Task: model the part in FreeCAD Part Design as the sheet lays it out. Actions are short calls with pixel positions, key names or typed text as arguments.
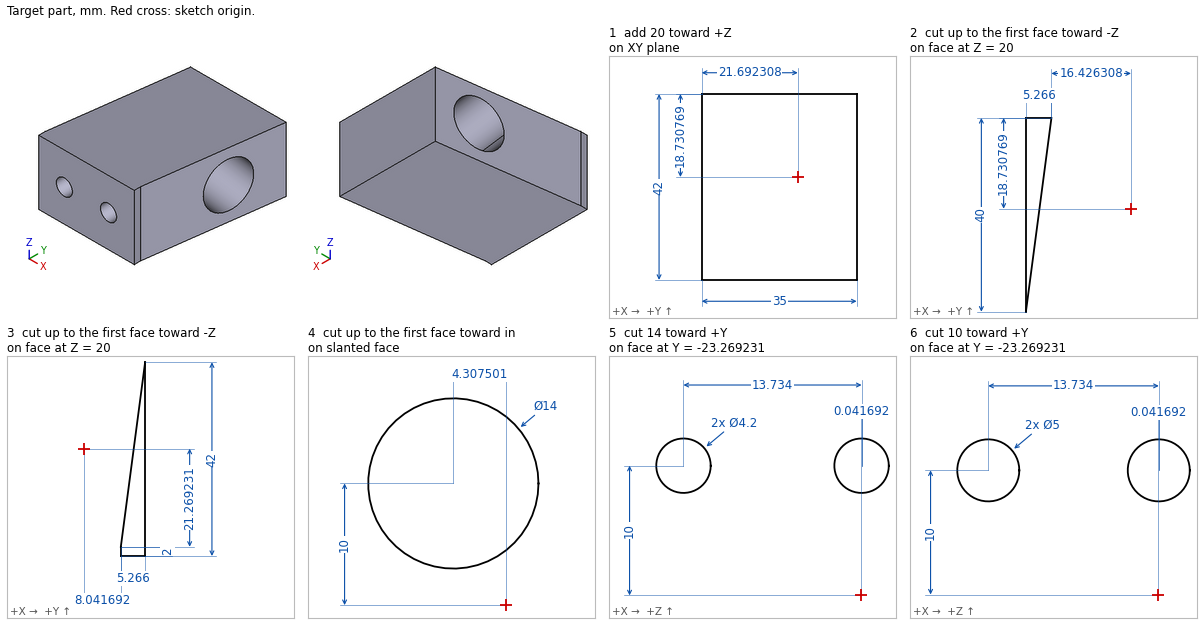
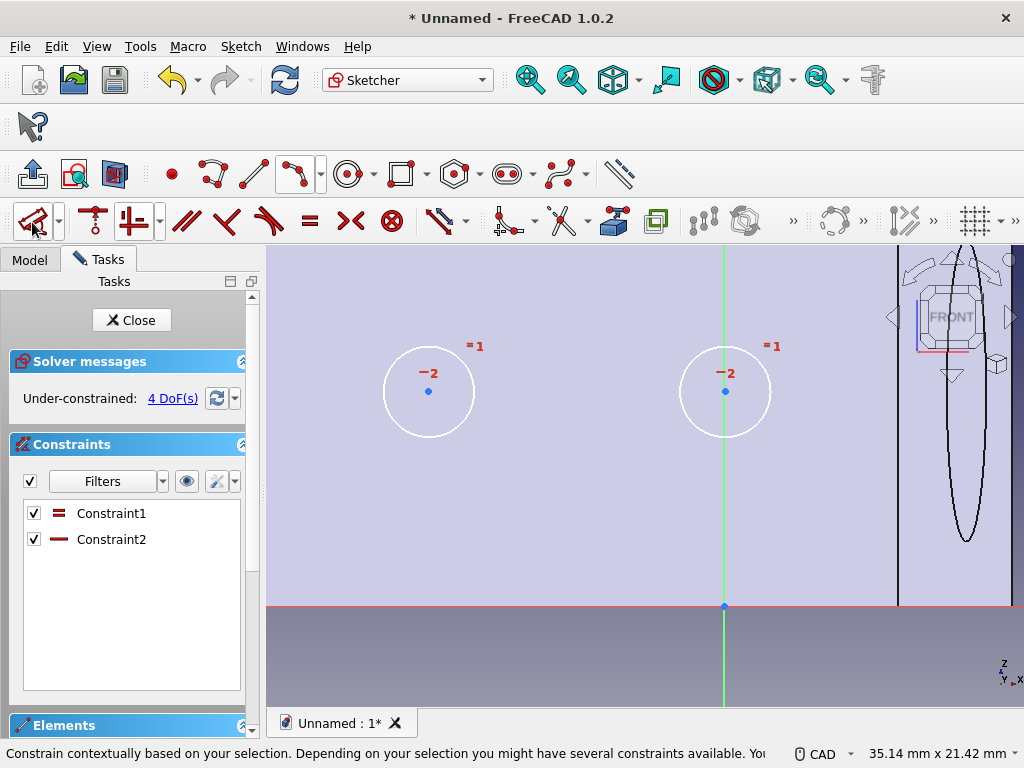
click(461, 360)
click(484, 337)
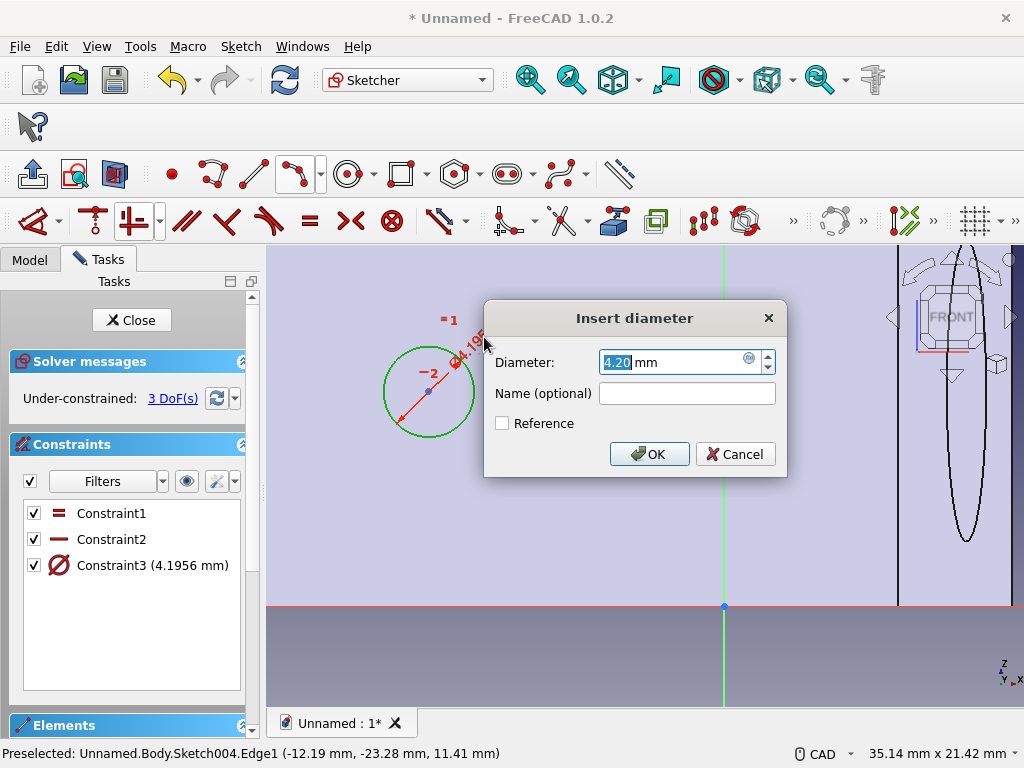
text(4.2)
key(Return)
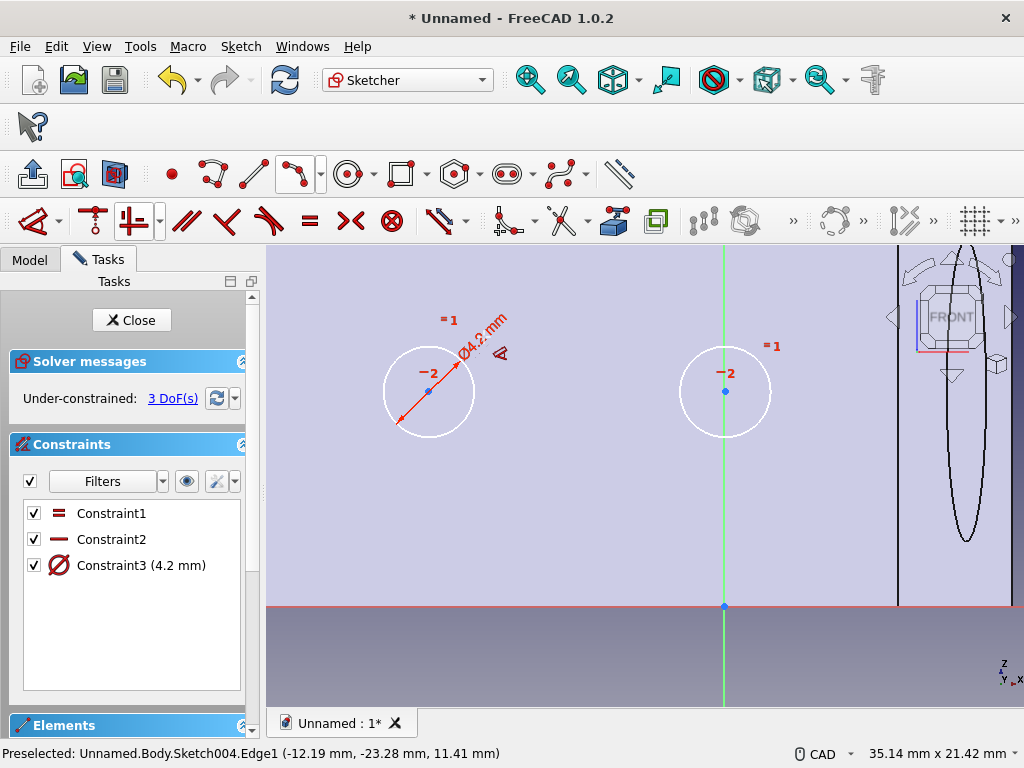
click(429, 392)
click(395, 499)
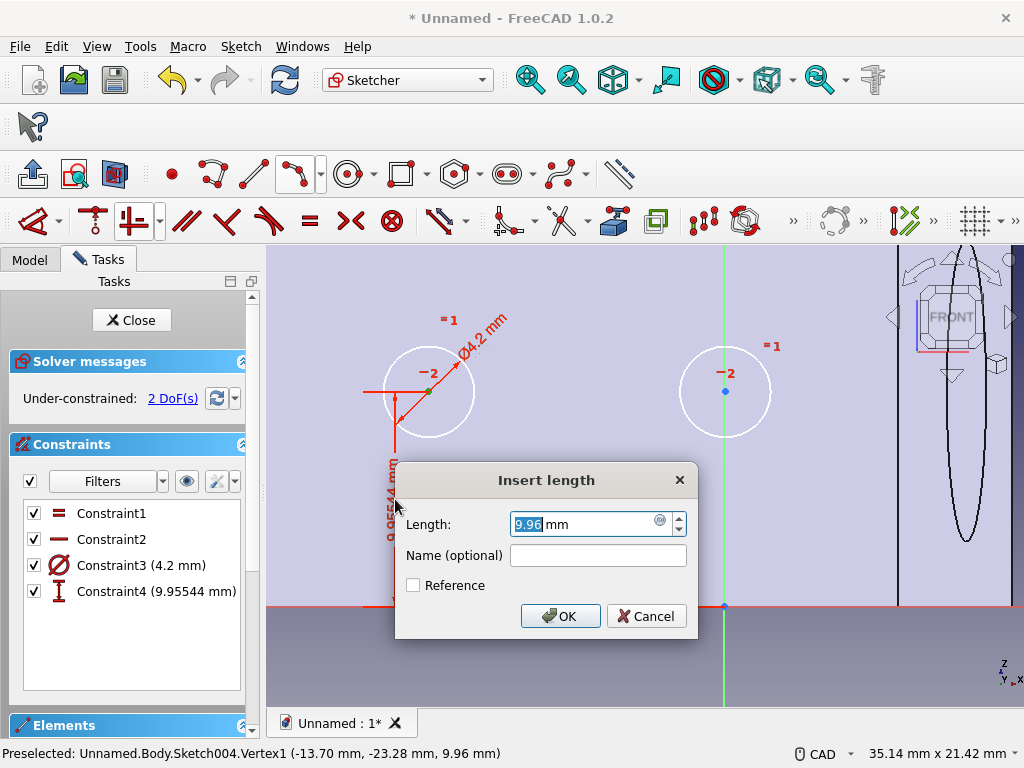
text(10)
key(Return)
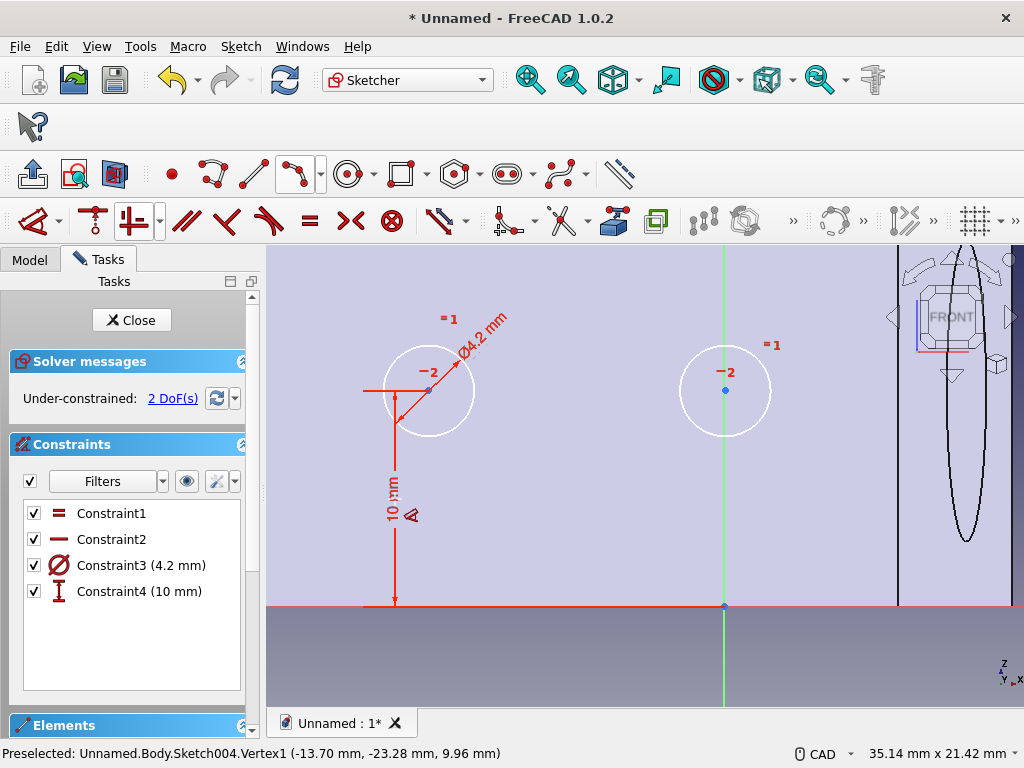
click(429, 391)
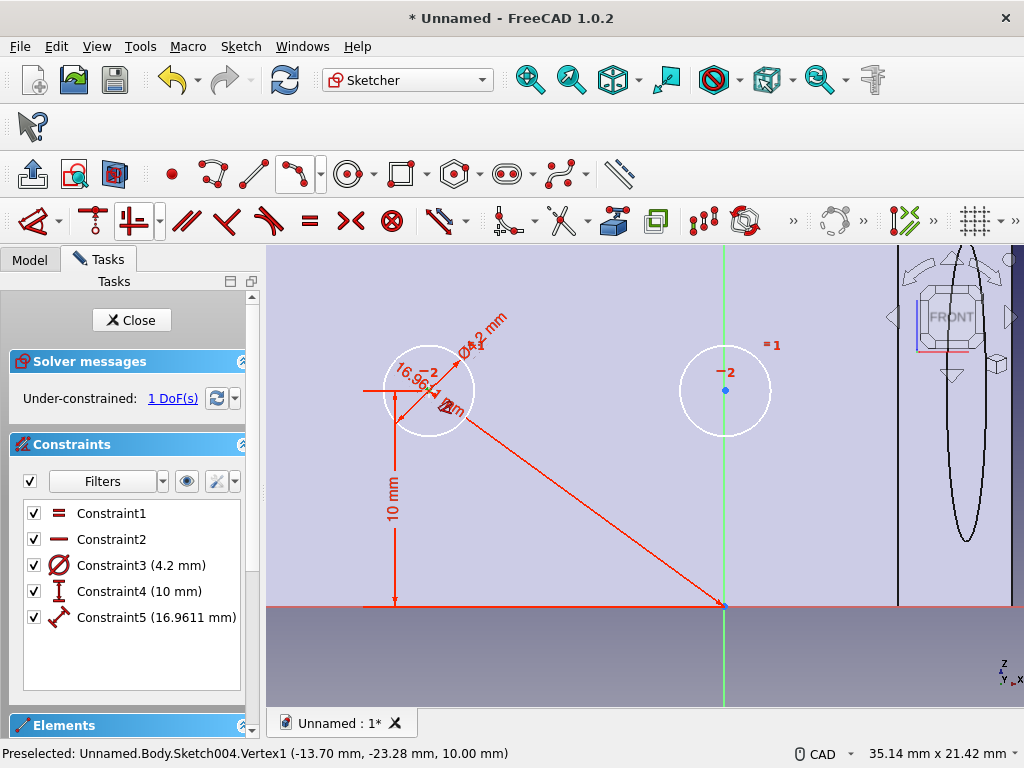
click(725, 391)
click(577, 357)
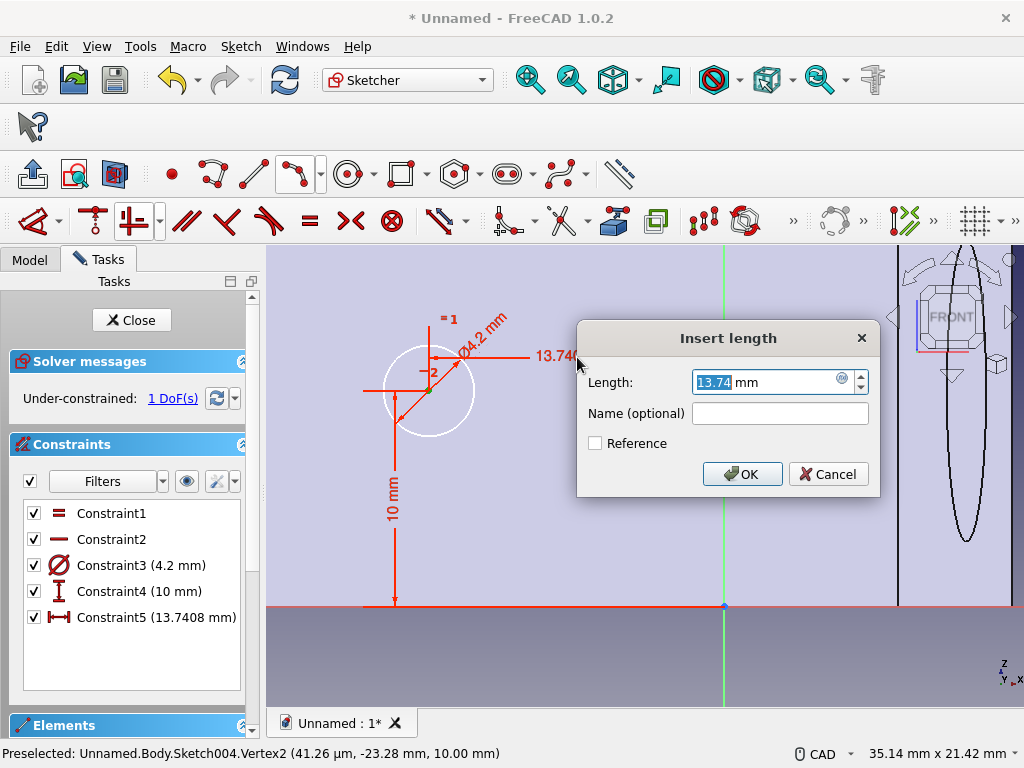
text(13.734)
key(Return)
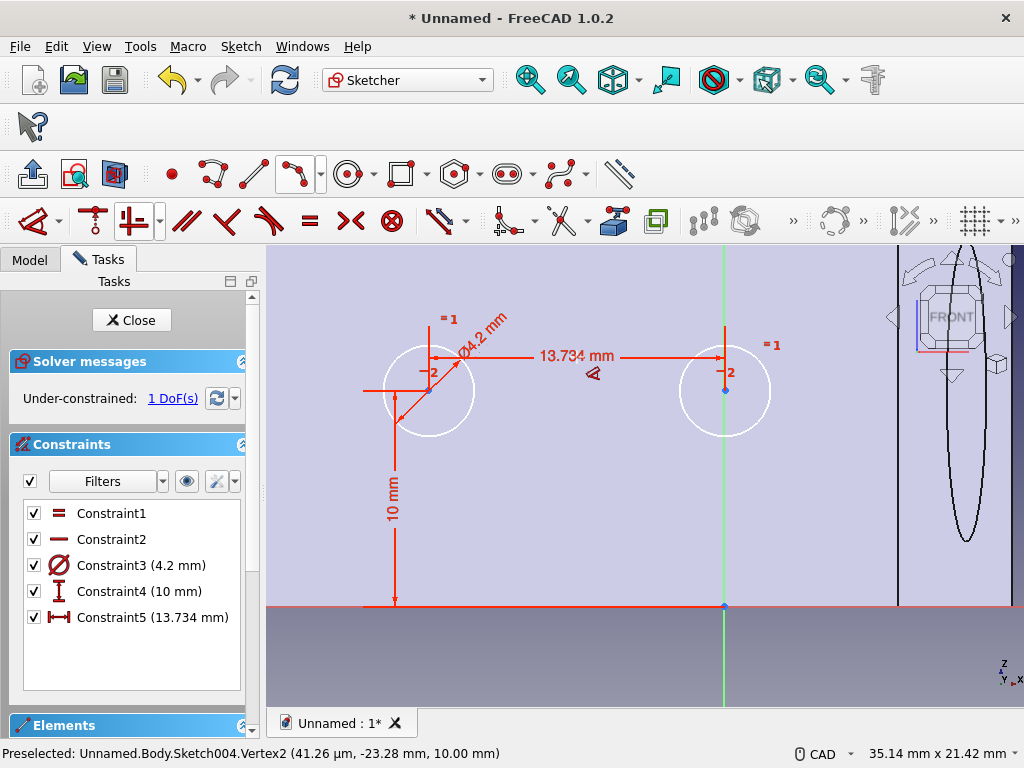
scroll(725, 391, up, 19)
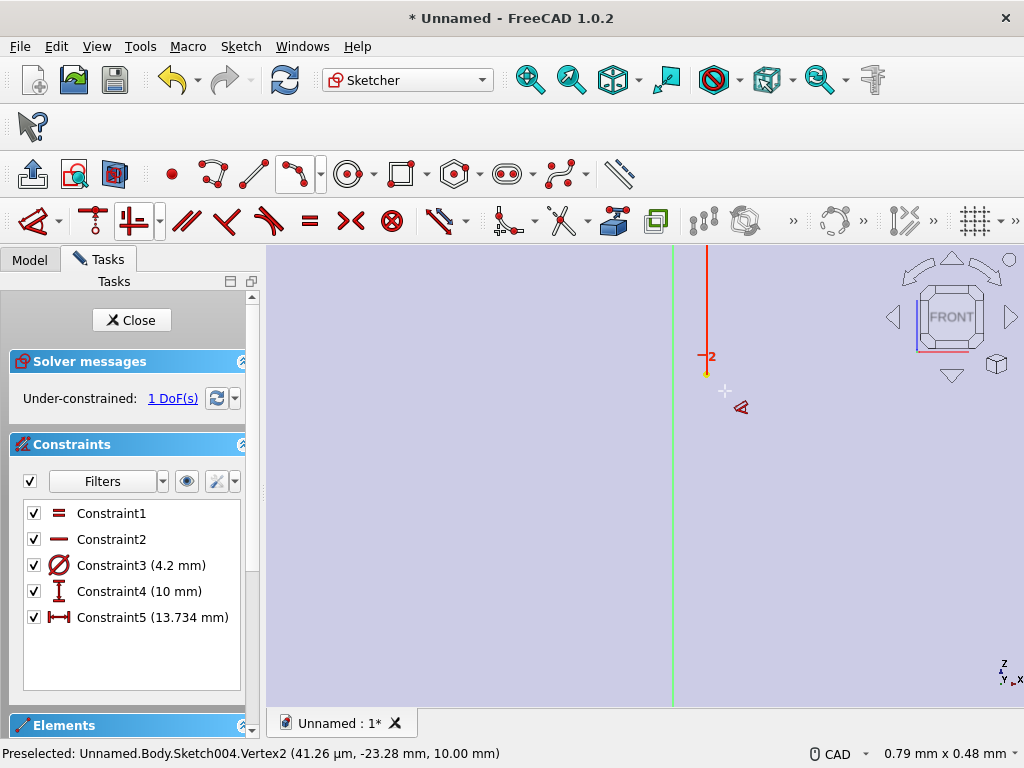
click(707, 375)
click(690, 341)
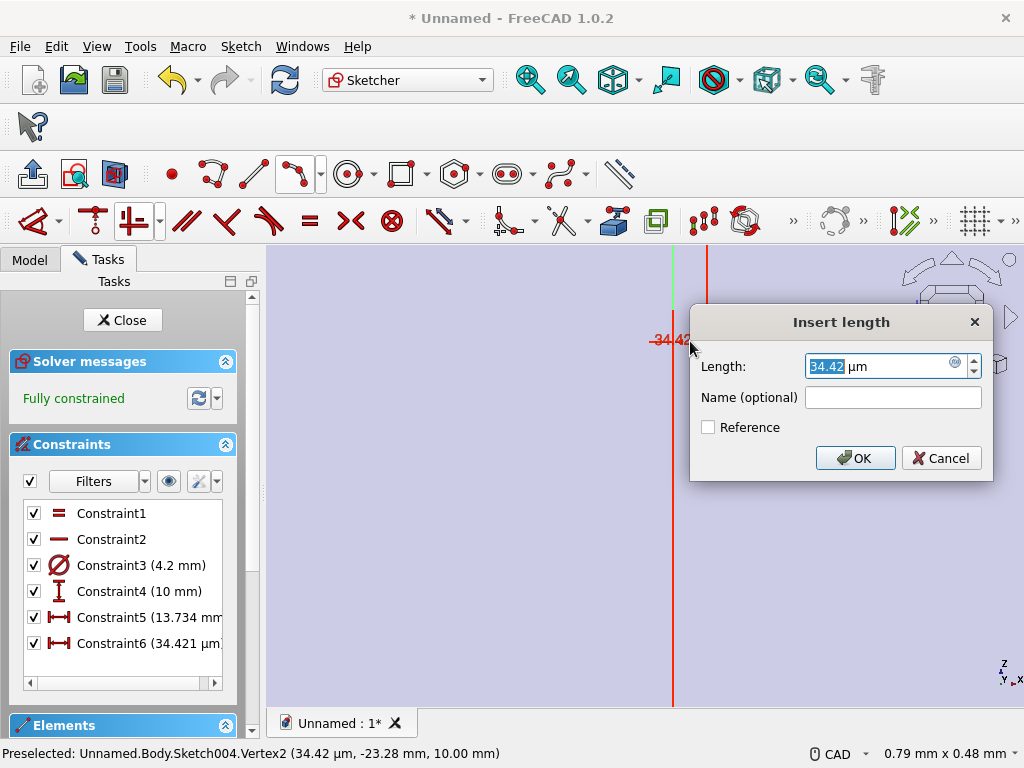
key(ctrl+a)
text(0.041692 mm)
key(Return)
key(Escape)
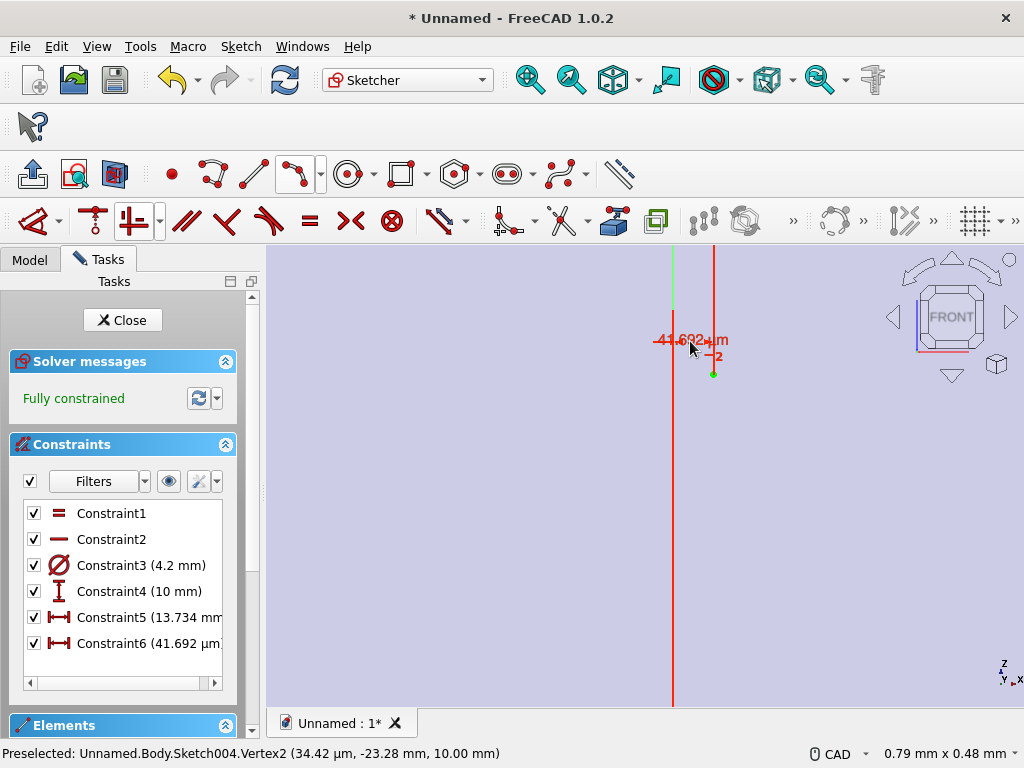
click(123, 320)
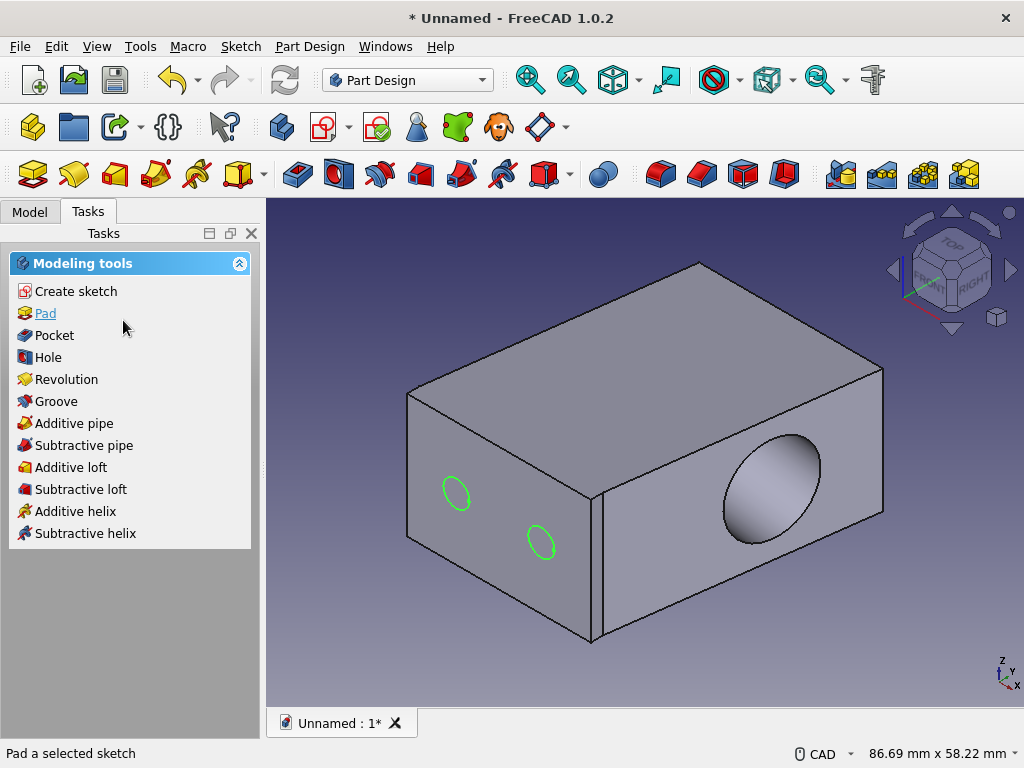
click(298, 174)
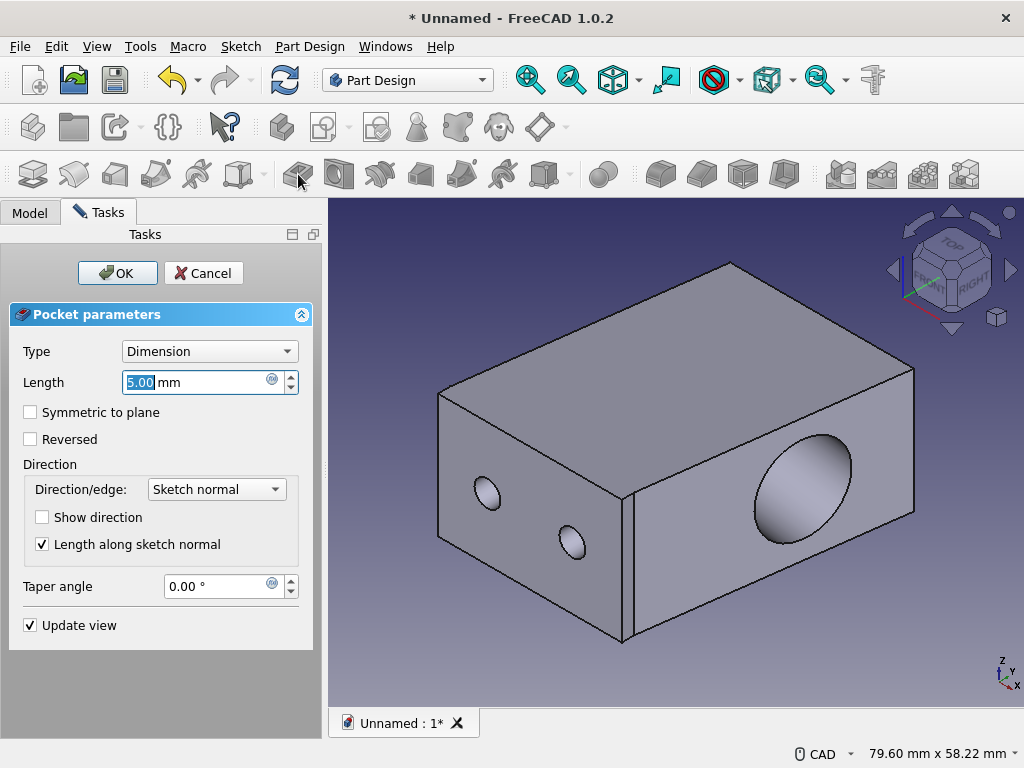
text(14)
key(Tab)